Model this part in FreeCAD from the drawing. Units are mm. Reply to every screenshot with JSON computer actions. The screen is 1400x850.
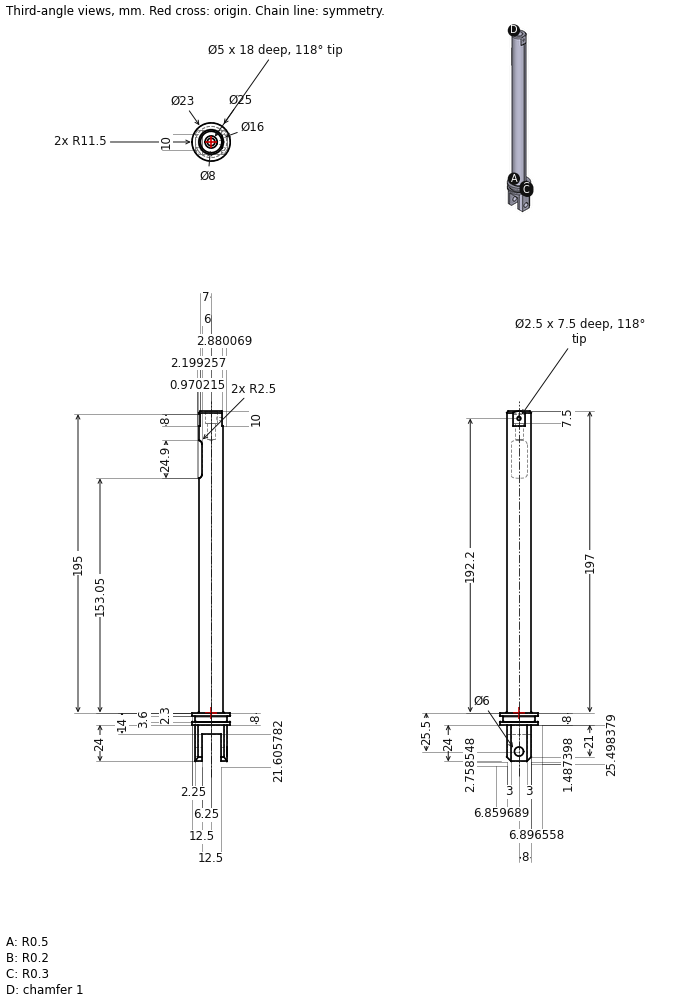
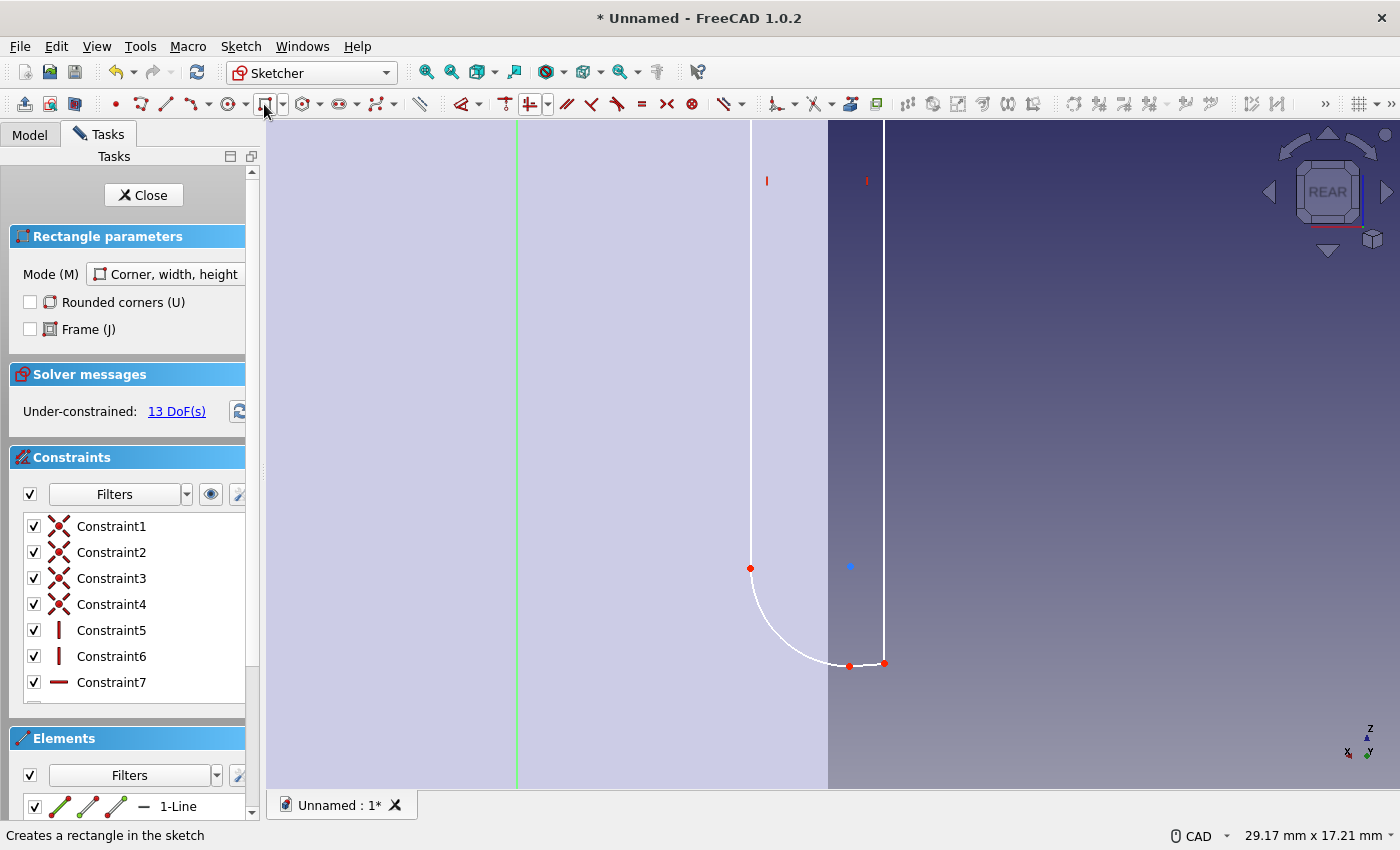
{"action": "scroll", "coordinate": [848, 666], "scroll_direction": "down", "scroll_amount": 7}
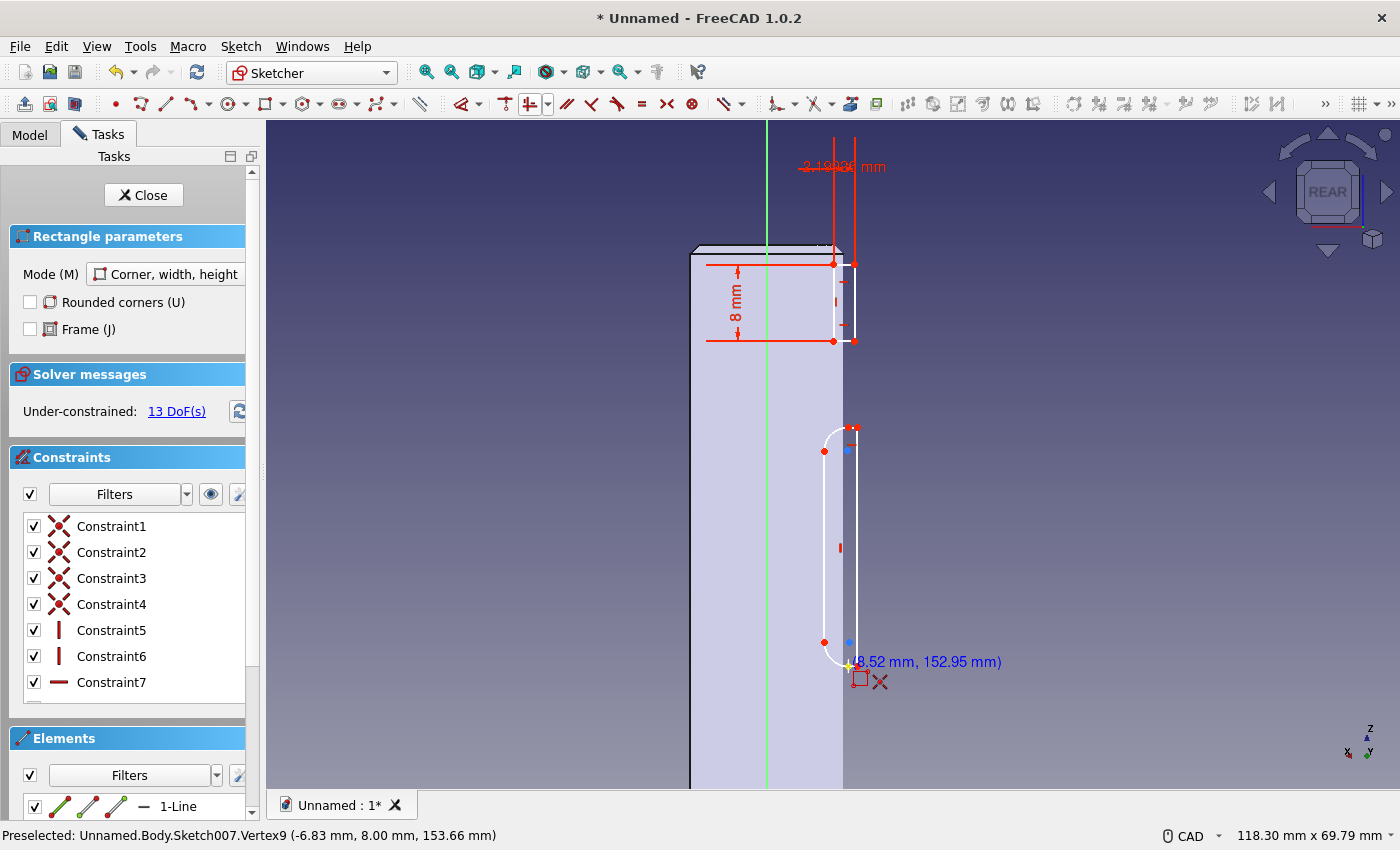
{"action": "left_click", "coordinate": [672, 245]}
{"action": "mouse_move", "coordinate": [700, 340]}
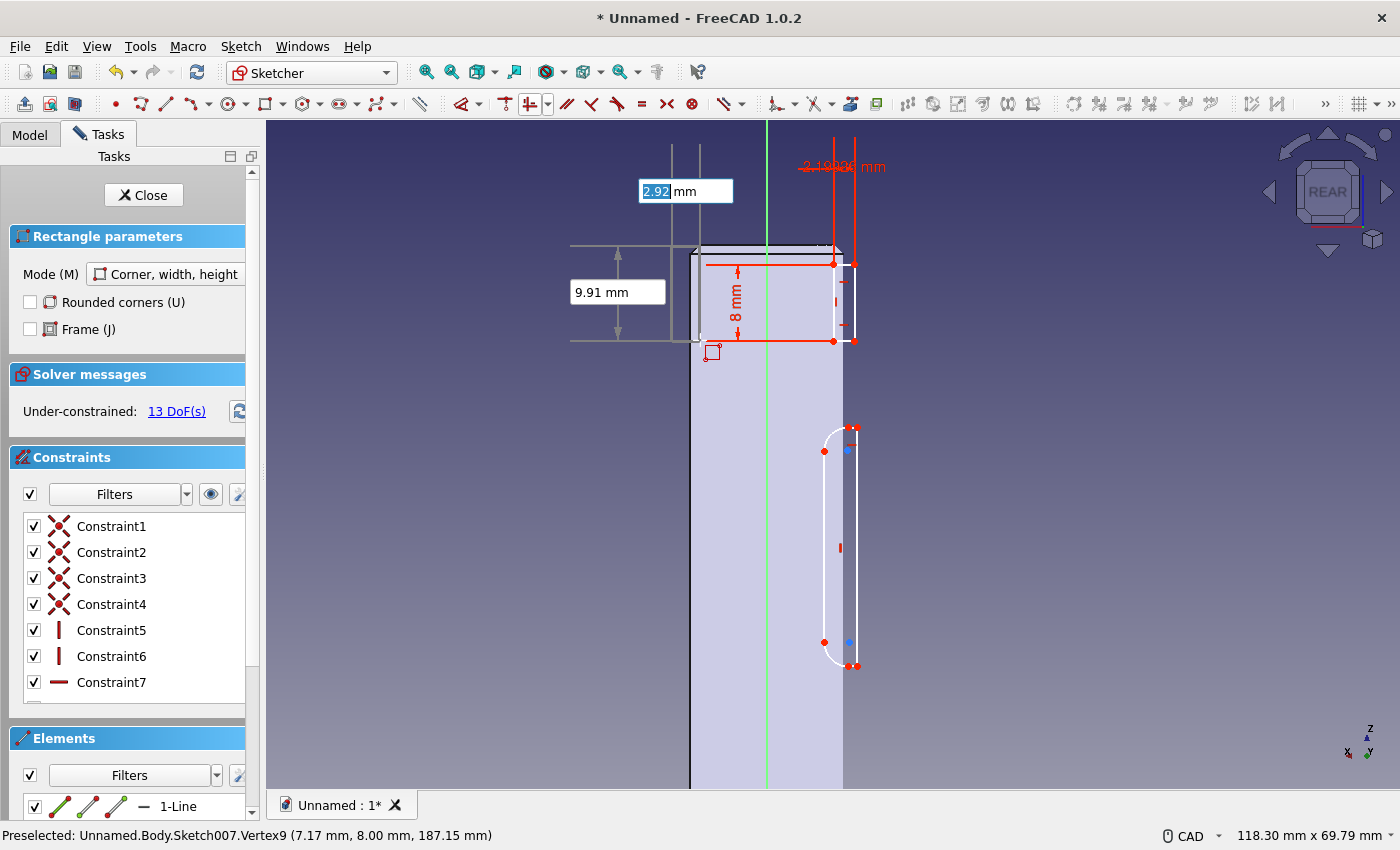
{"action": "type", "text": "2.880069"}
{"action": "key", "text": "Tab"}
{"action": "type", "text": "10"}
{"action": "key", "text": "Return"}
{"action": "key", "text": "Escape"}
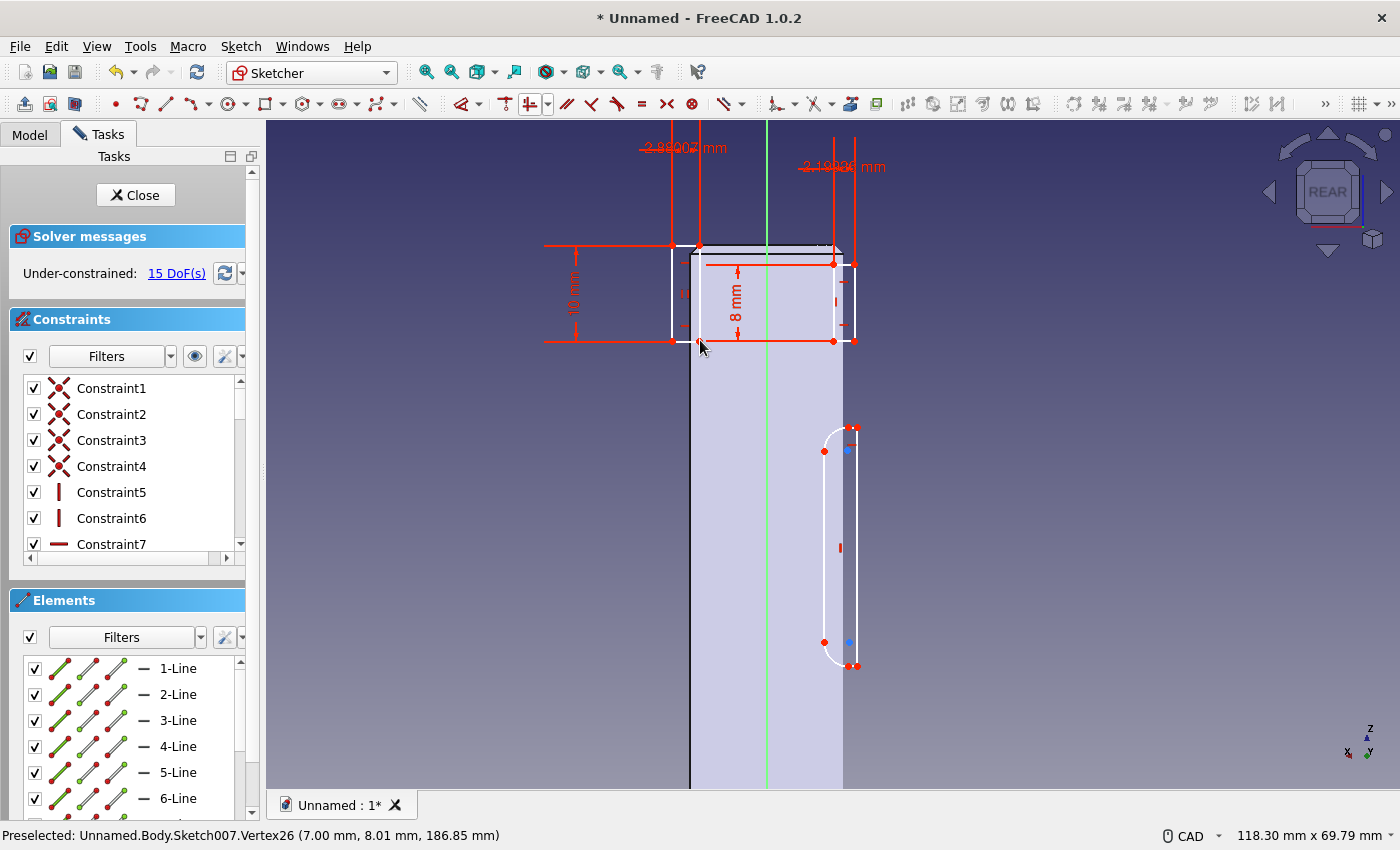
{"action": "scroll", "coordinate": [853, 666], "scroll_direction": "up", "scroll_amount": 6}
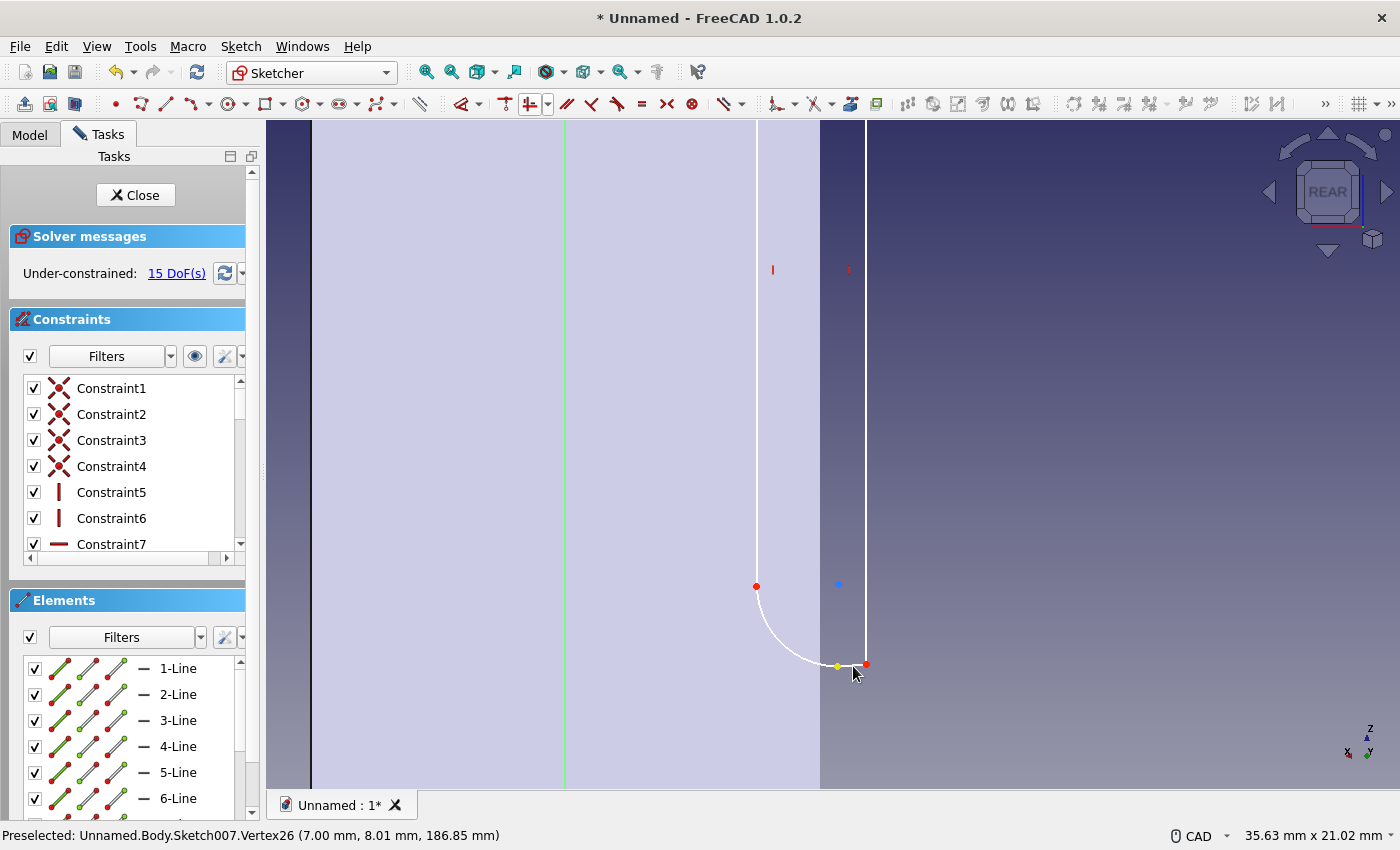
{"action": "left_click", "coordinate": [852, 666]}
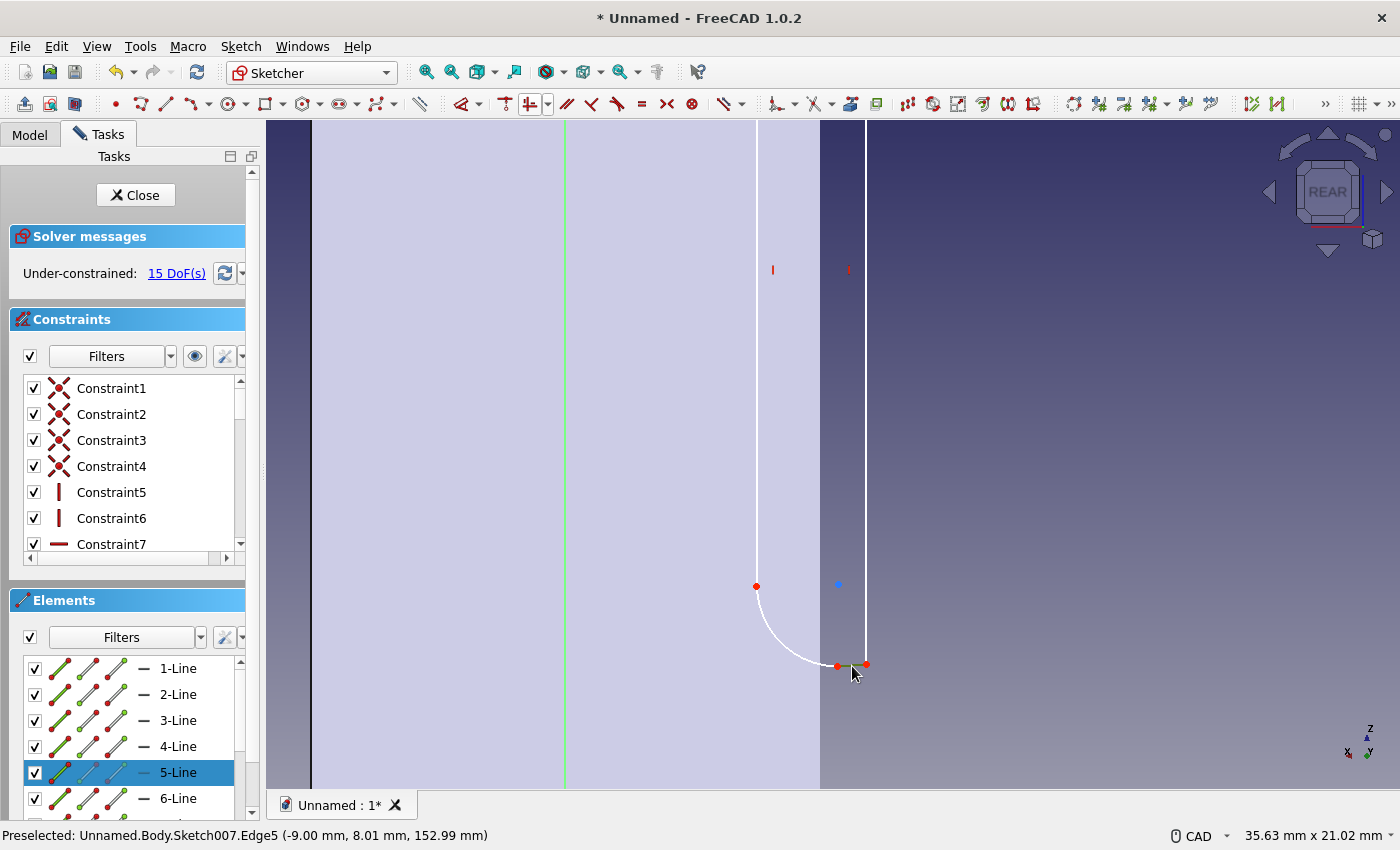
{"action": "left_click", "coordinate": [766, 622]}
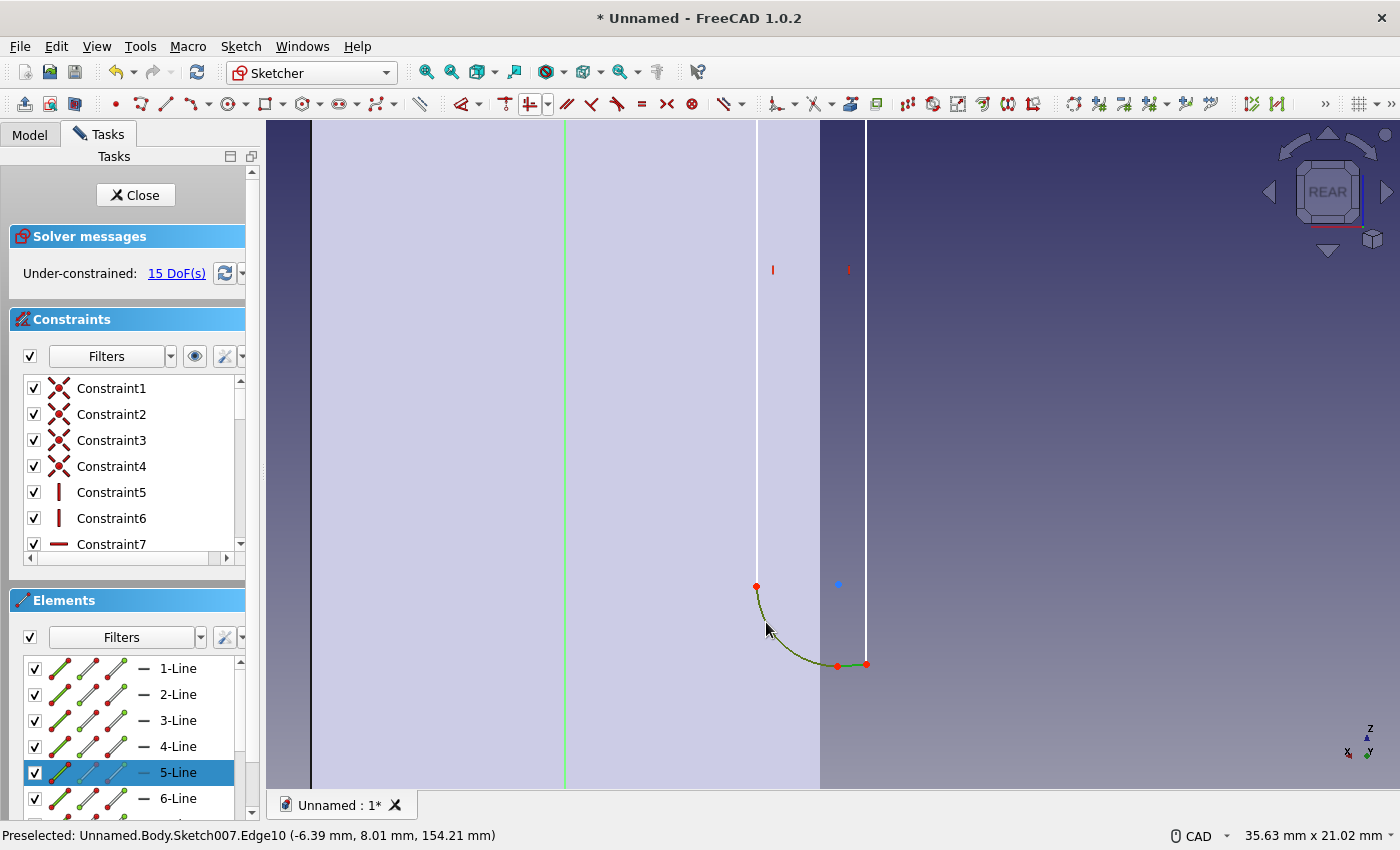
{"action": "left_click", "coordinate": [617, 104]}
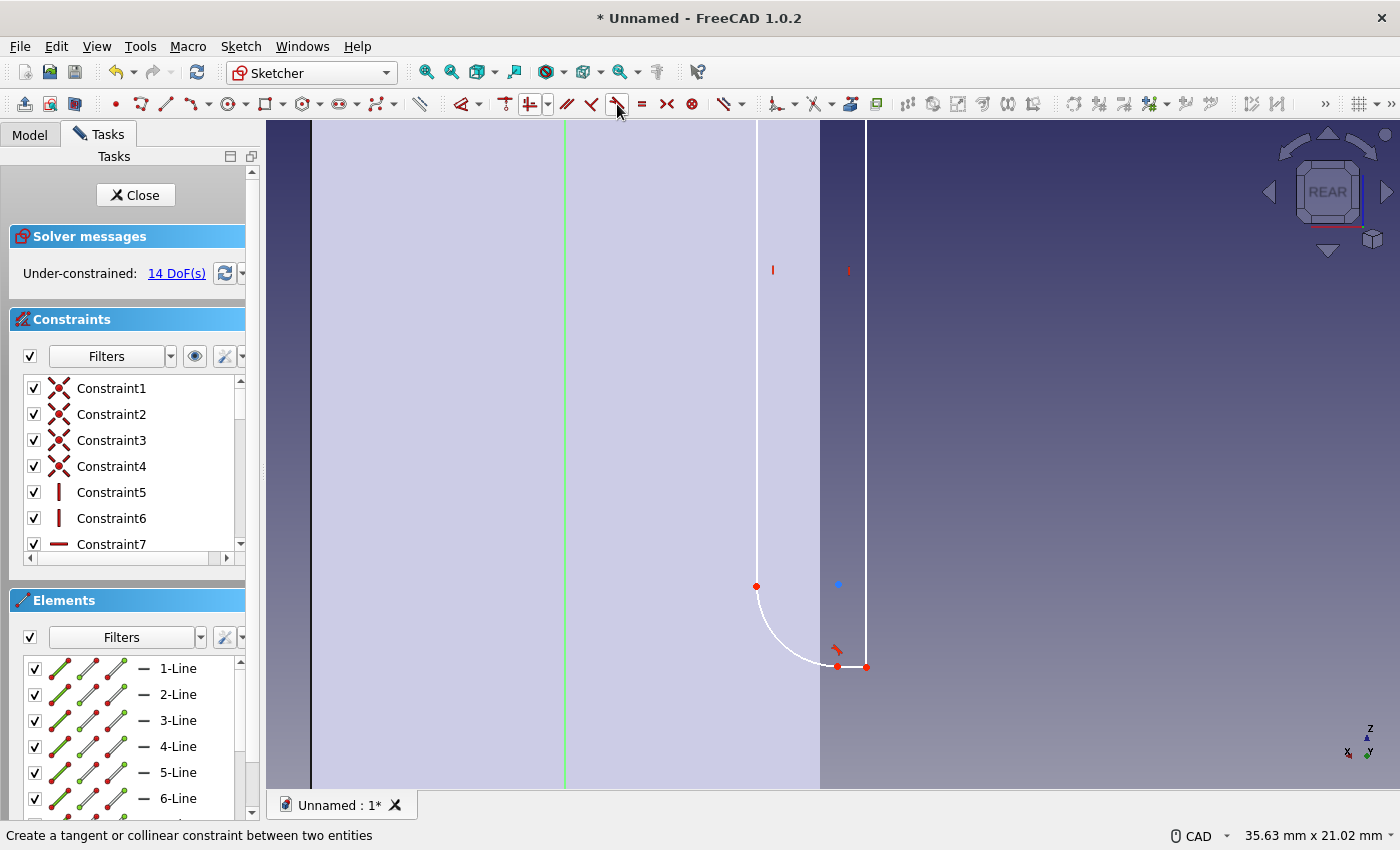
{"action": "scroll", "coordinate": [853, 666], "scroll_direction": "down", "scroll_amount": 6}